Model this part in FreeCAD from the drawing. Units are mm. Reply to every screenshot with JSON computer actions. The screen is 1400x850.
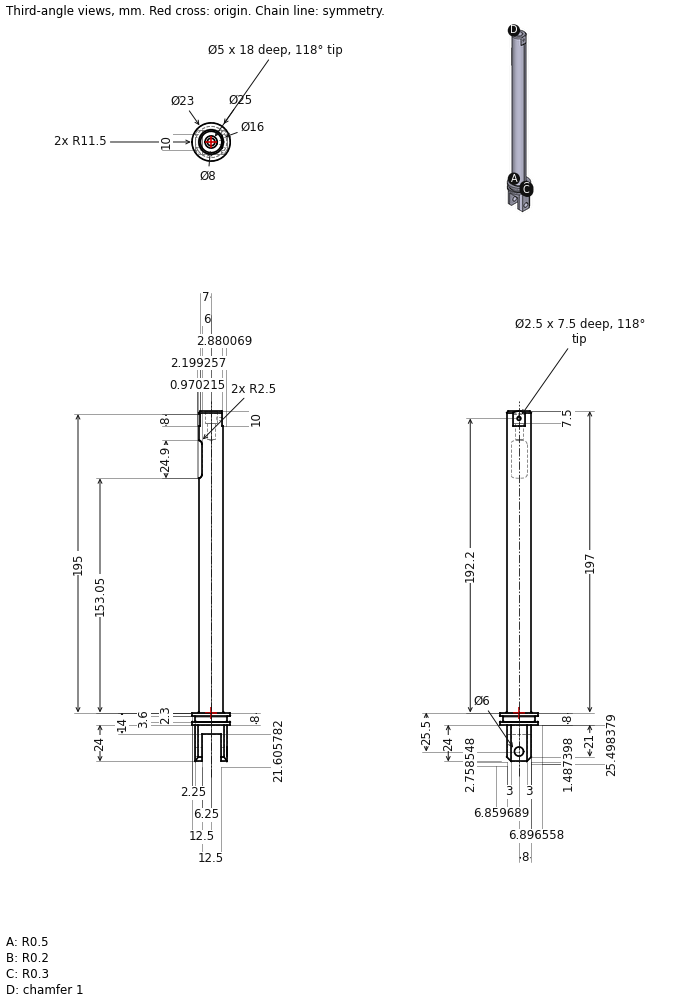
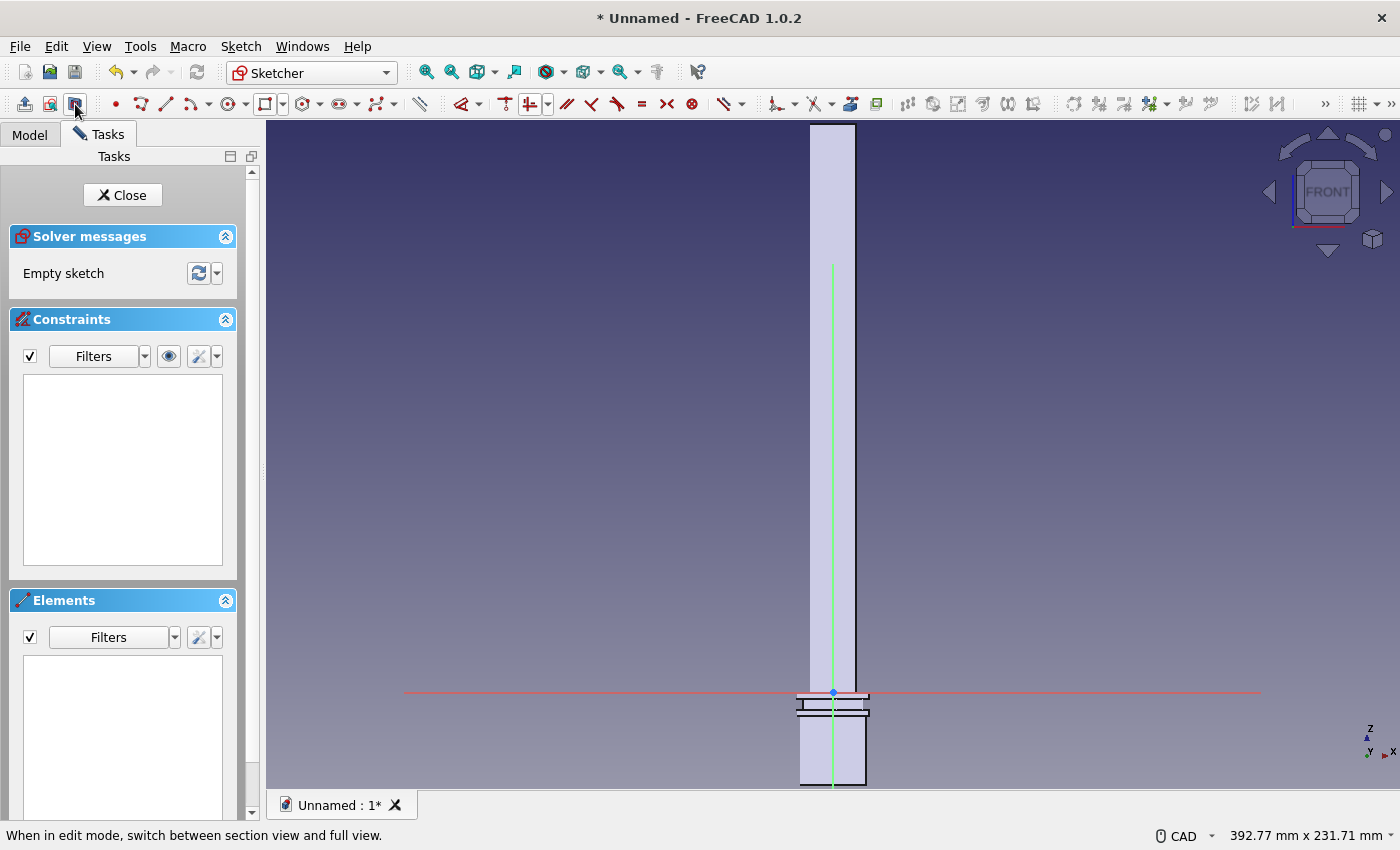
{"action": "scroll", "coordinate": [764, 454], "scroll_direction": "down", "scroll_amount": 5}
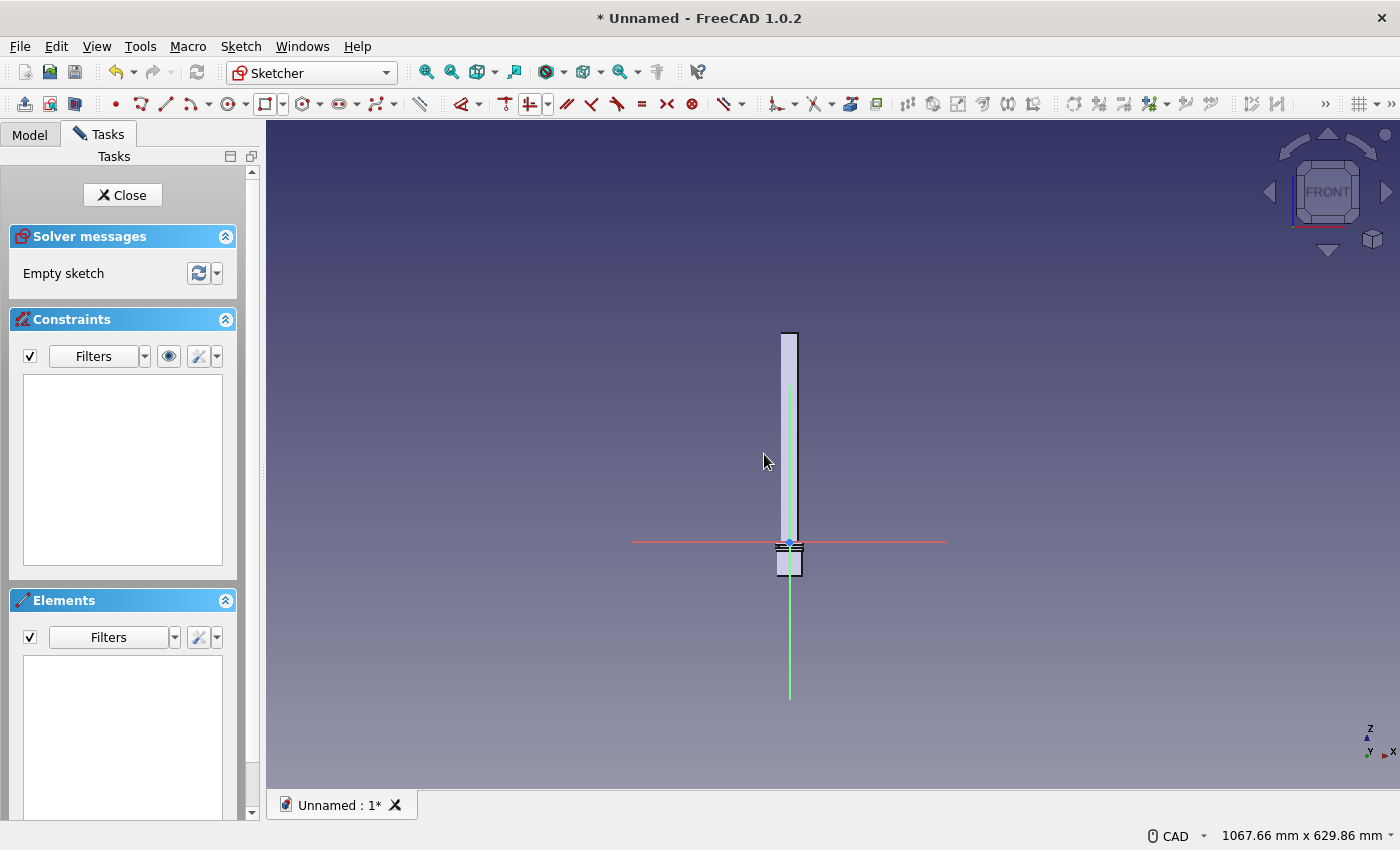
{"action": "scroll", "coordinate": [792, 572], "scroll_direction": "up", "scroll_amount": 12}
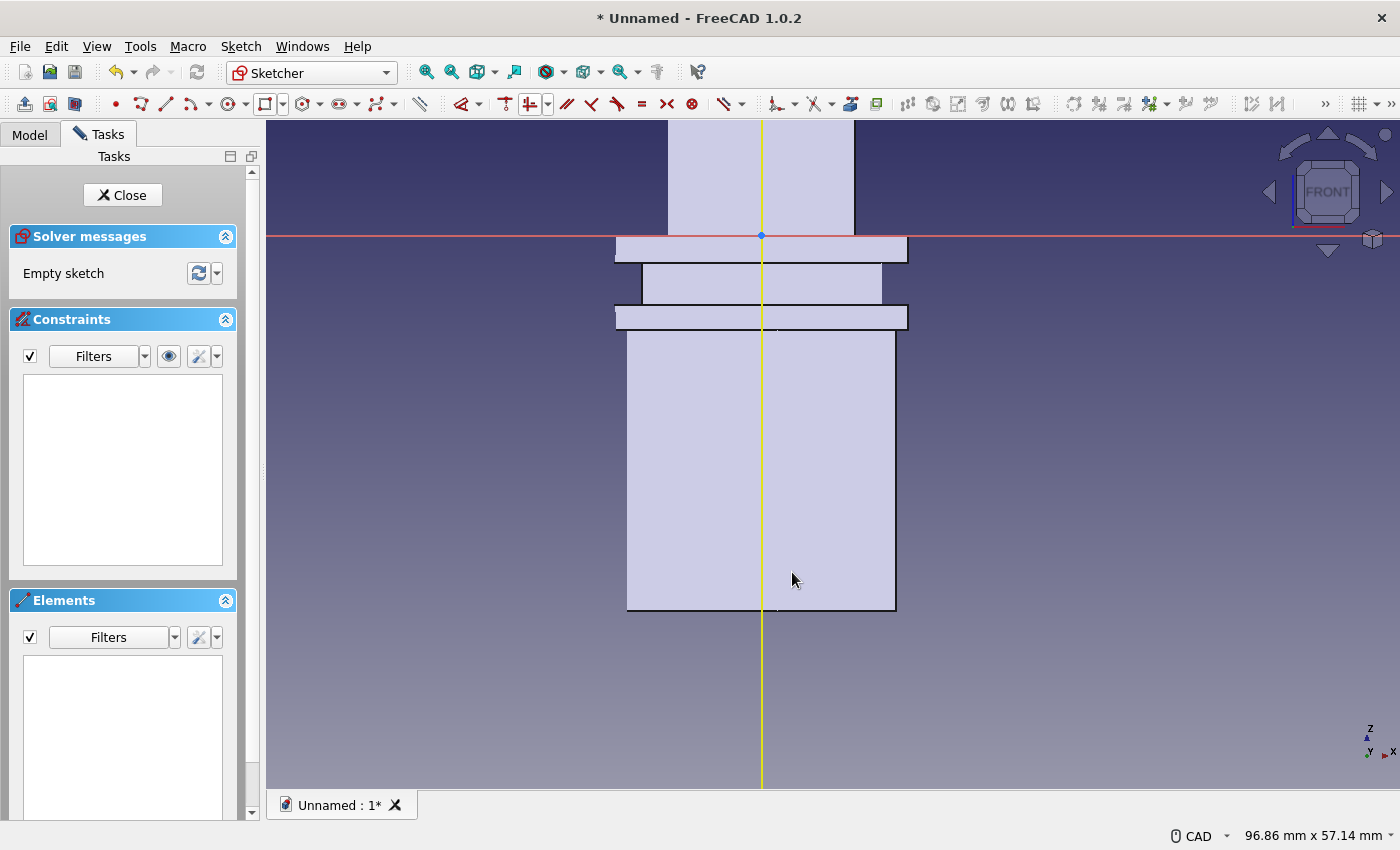
{"action": "left_click", "coordinate": [264, 104]}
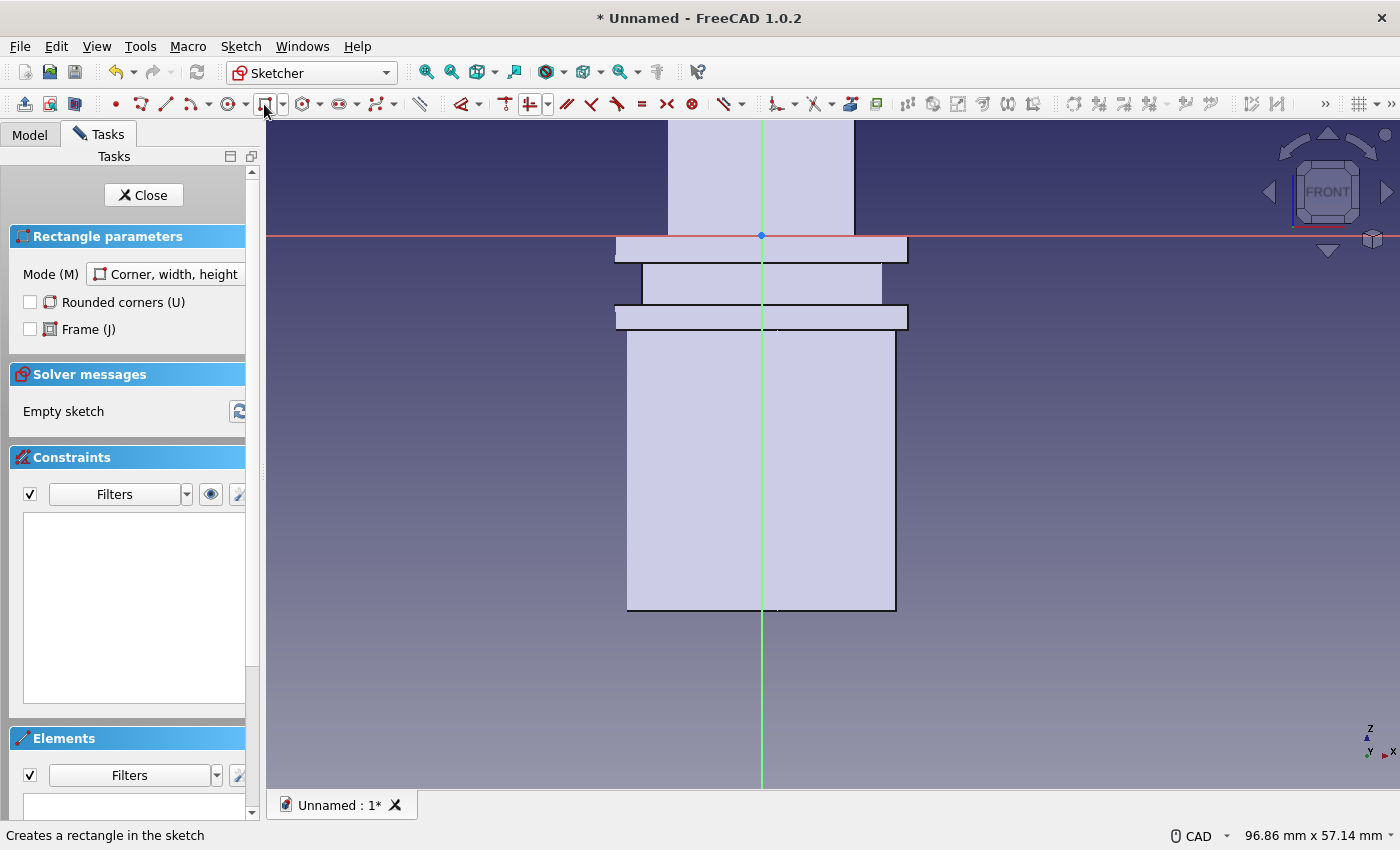
{"action": "left_click", "coordinate": [688, 400]}
{"action": "mouse_move", "coordinate": [835, 653]}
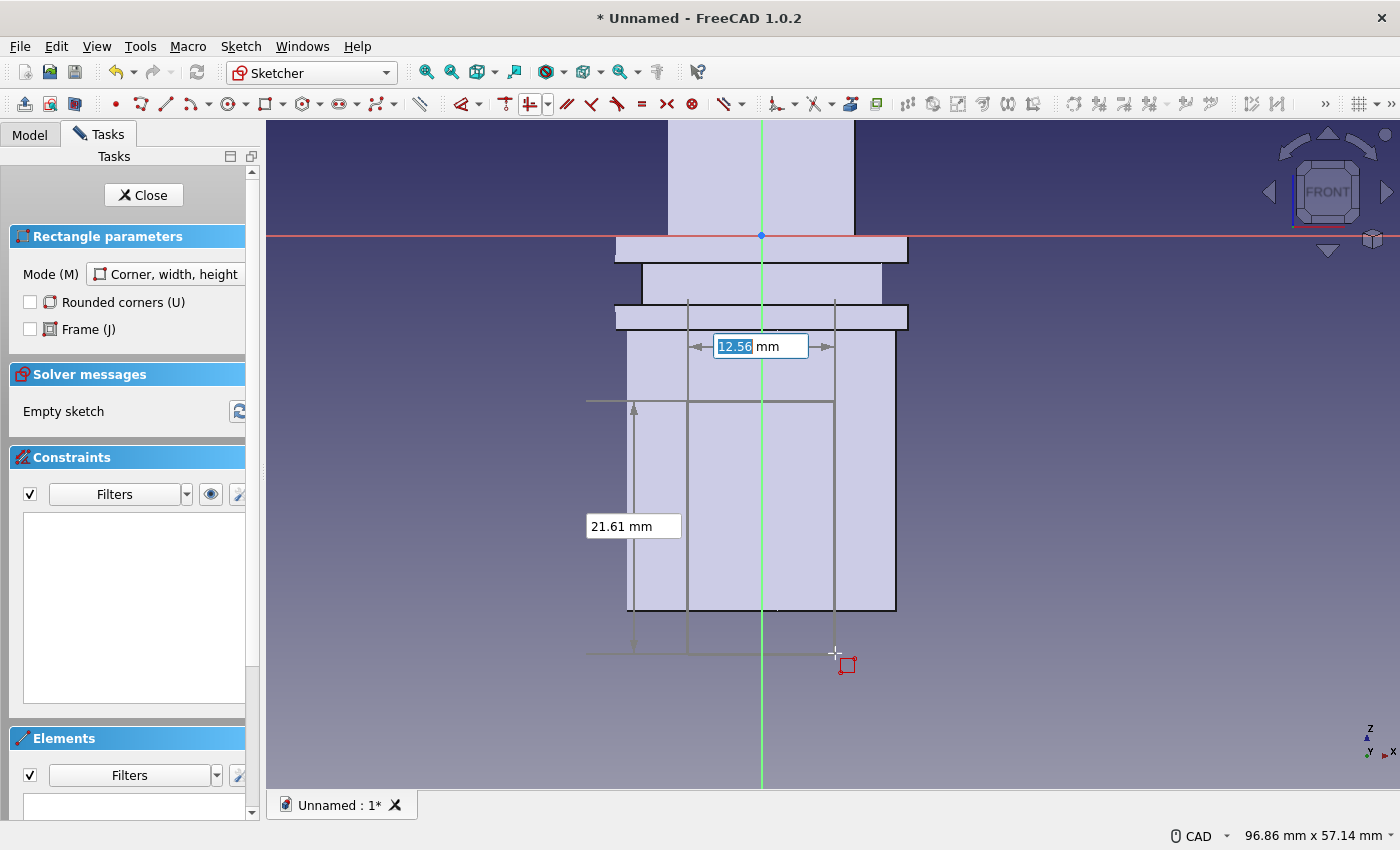
{"action": "type", "text": "12.5"}
{"action": "key", "text": "Tab"}
{"action": "type", "text": "21.605782"}
{"action": "key", "text": "Return"}
{"action": "key", "text": "Escape"}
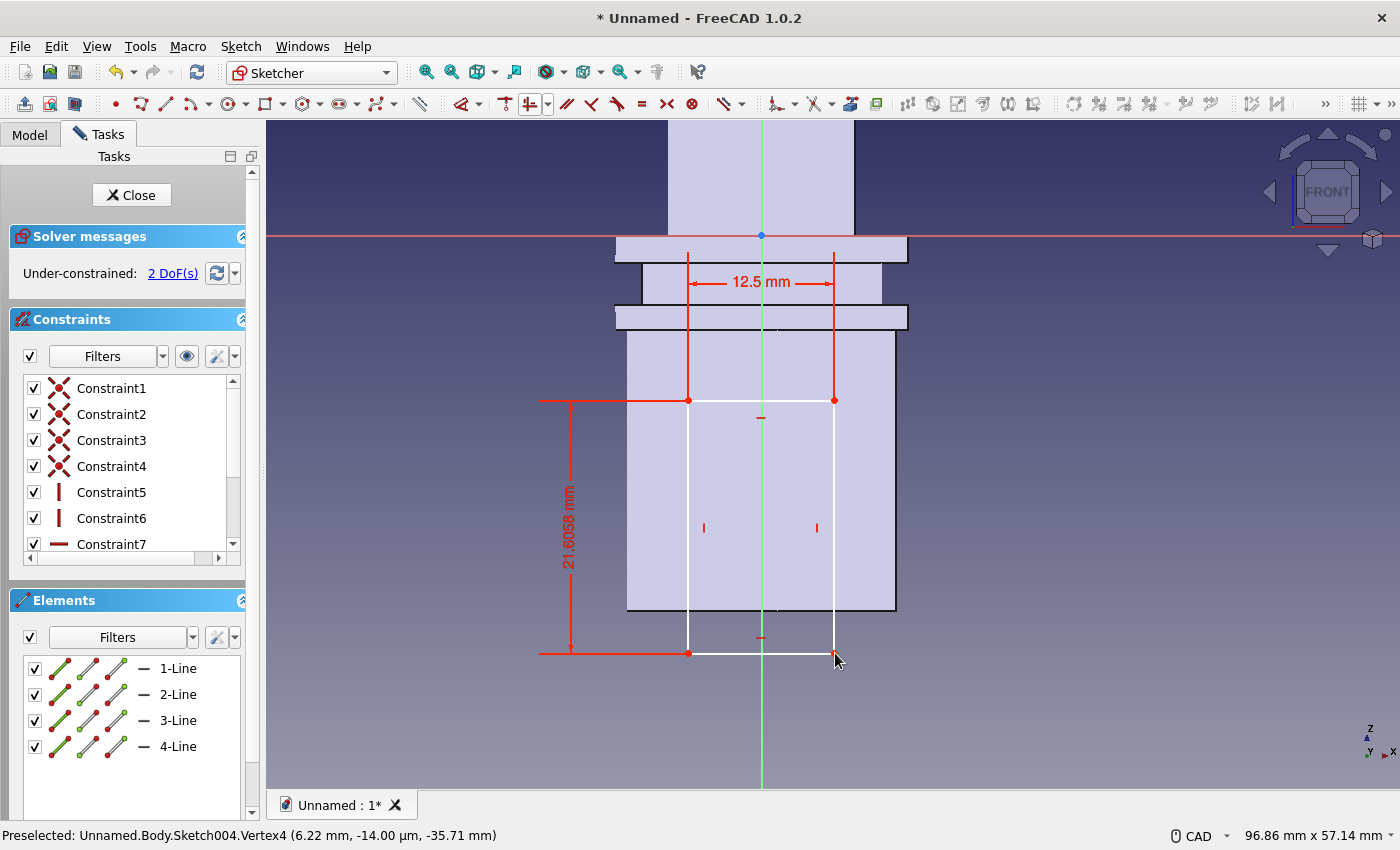
{"action": "left_click", "coordinate": [460, 104]}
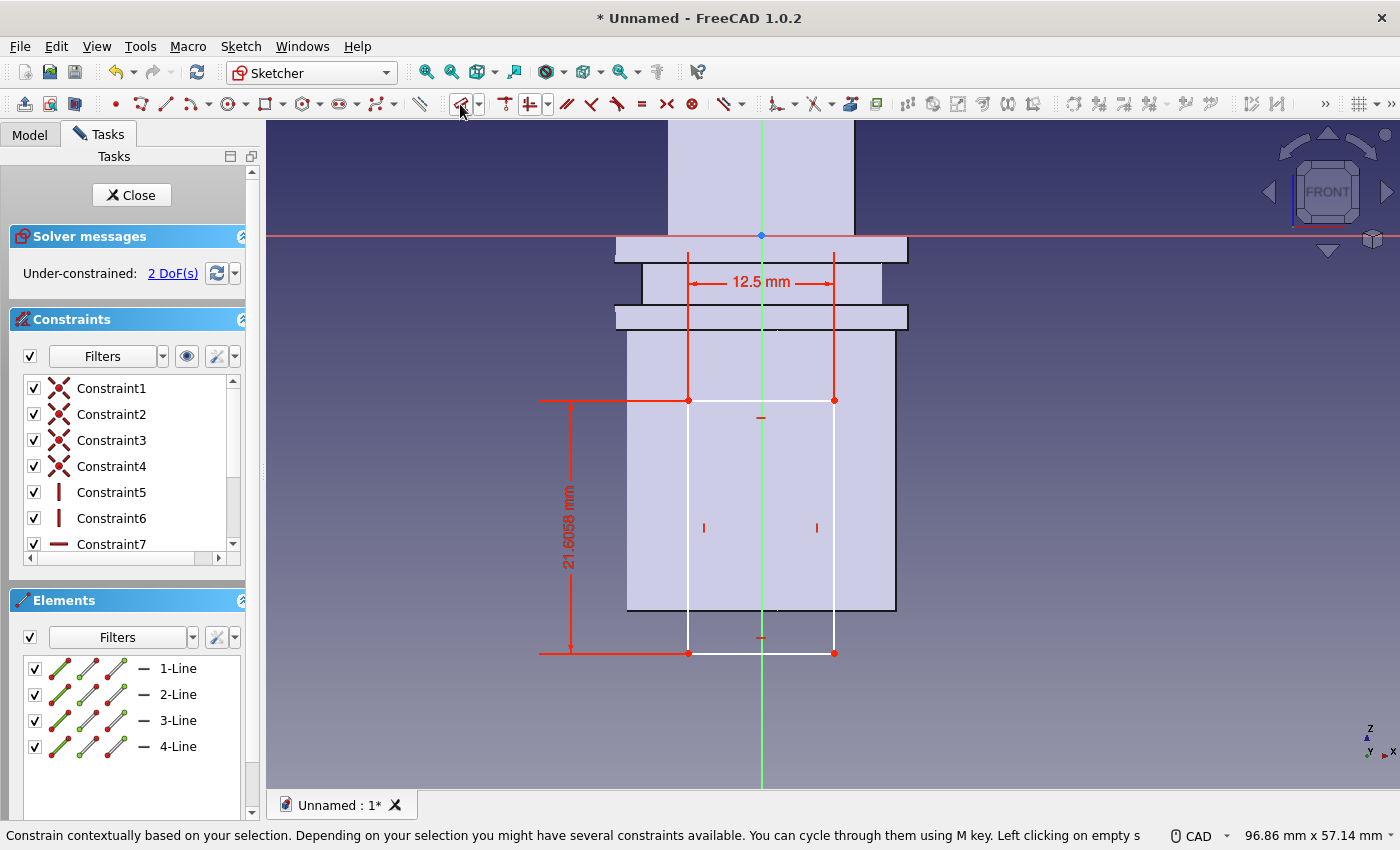
{"action": "left_click", "coordinate": [688, 401]}
{"action": "left_click", "coordinate": [654, 318]}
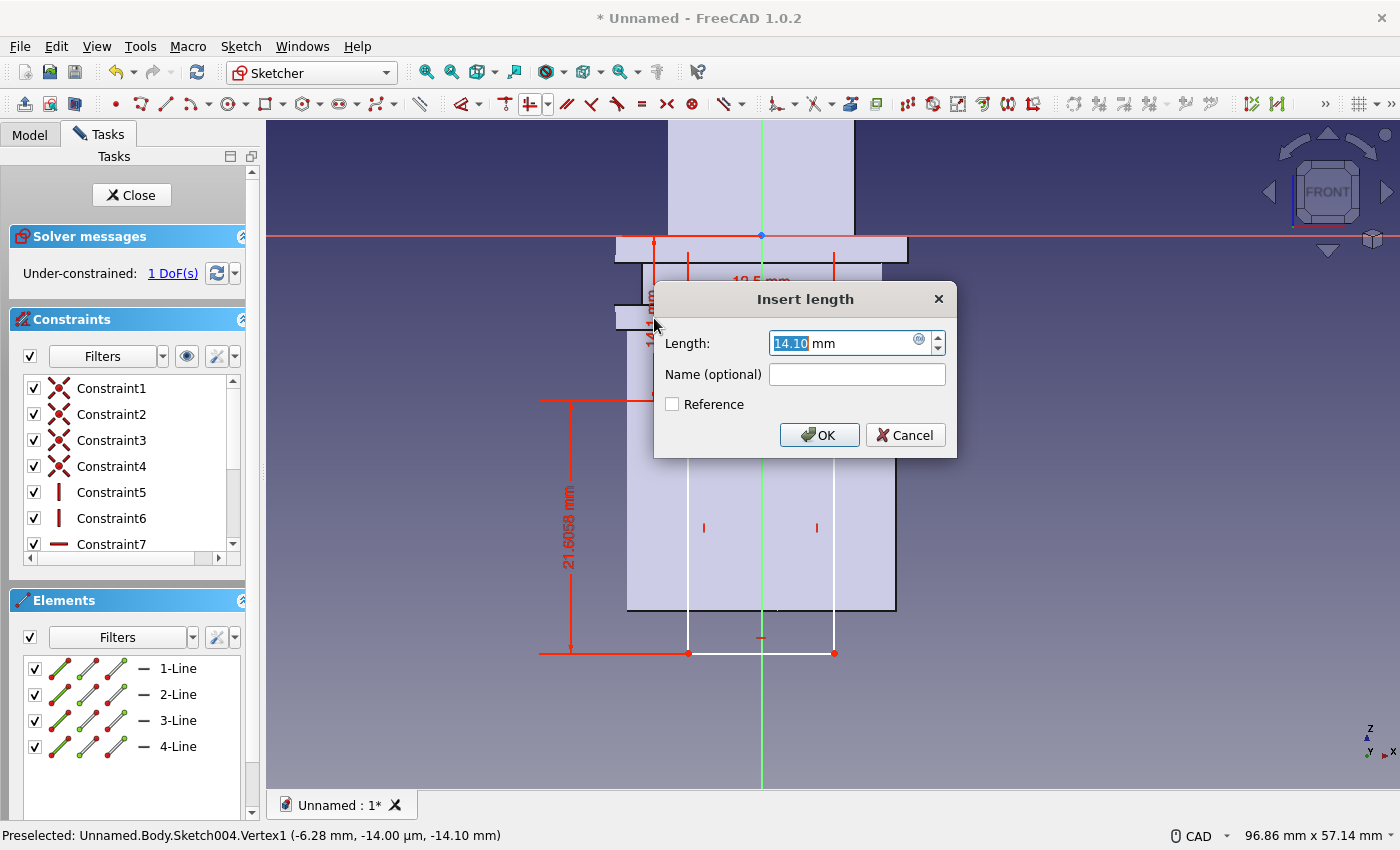
{"action": "type", "text": "14"}
{"action": "key", "text": "Return"}